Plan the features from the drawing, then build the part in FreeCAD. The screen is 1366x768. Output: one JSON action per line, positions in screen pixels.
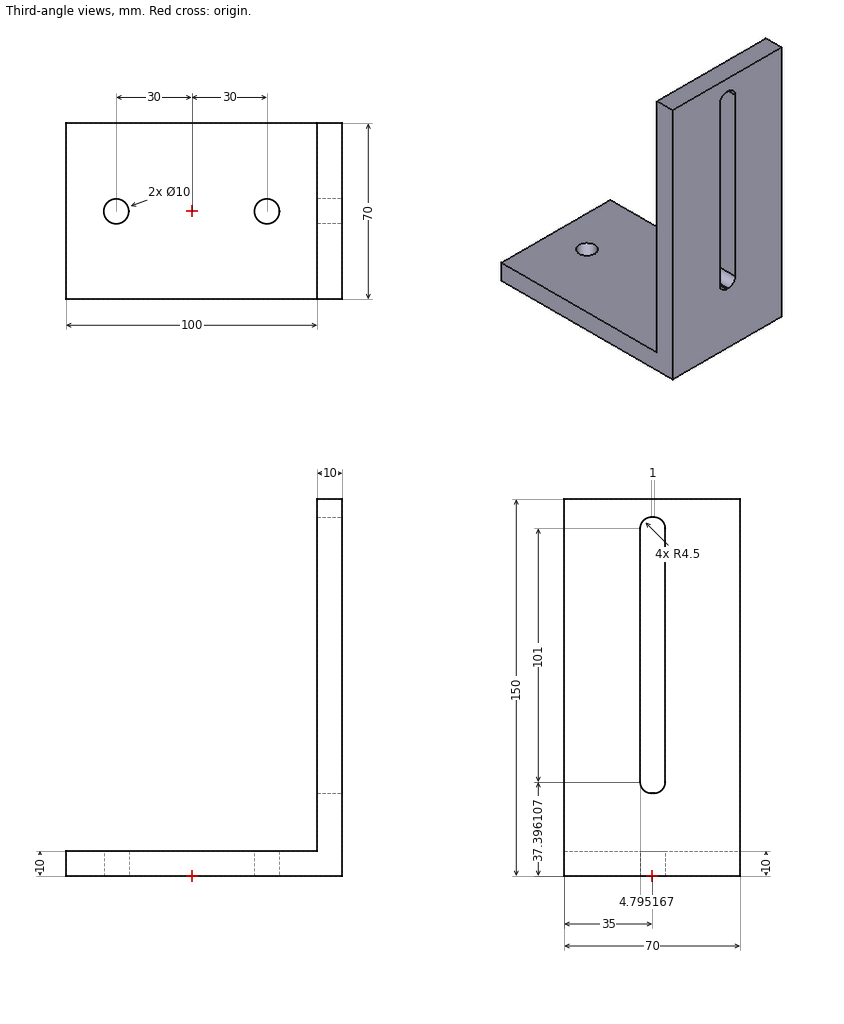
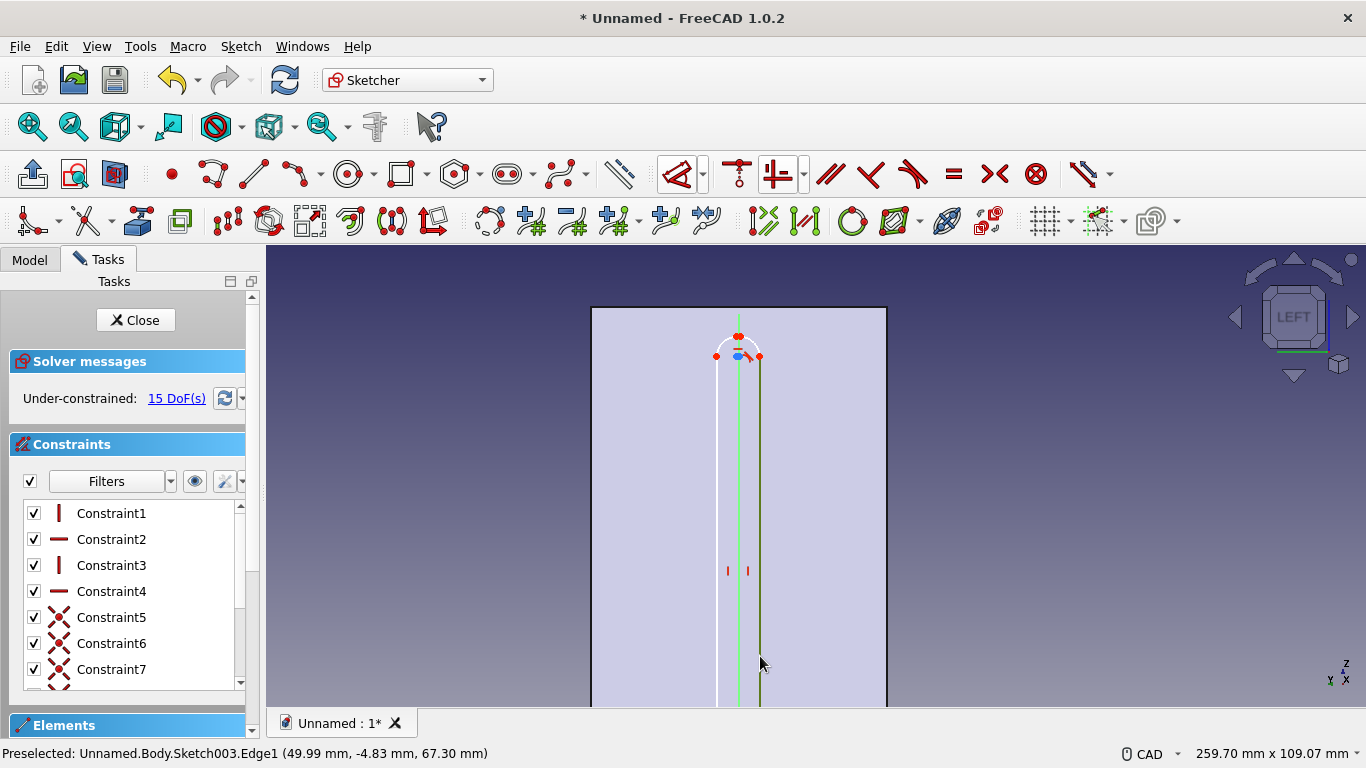
{"action": "scroll", "coordinate": [755, 343], "scroll_direction": "down", "scroll_amount": 4}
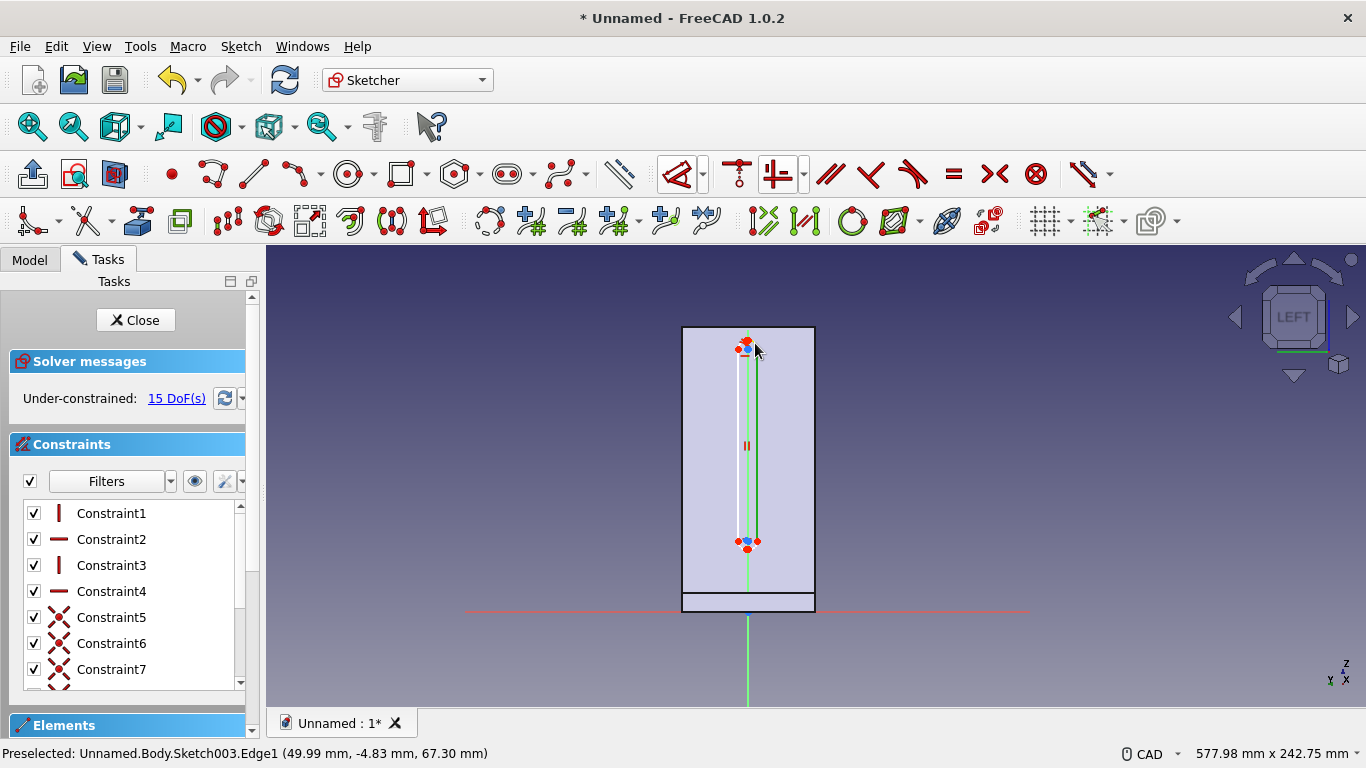
{"action": "scroll", "coordinate": [755, 547], "scroll_direction": "up", "scroll_amount": 4}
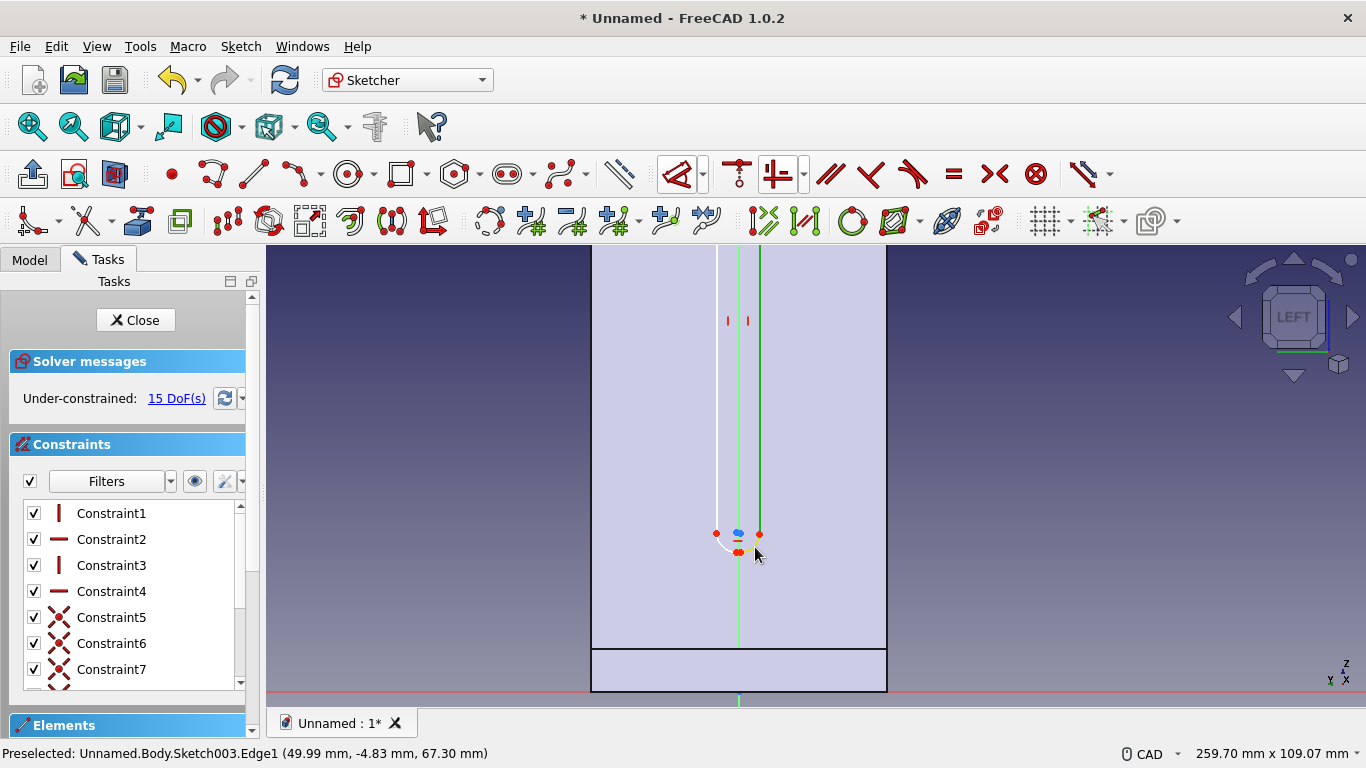
{"action": "left_click", "coordinate": [754, 547]}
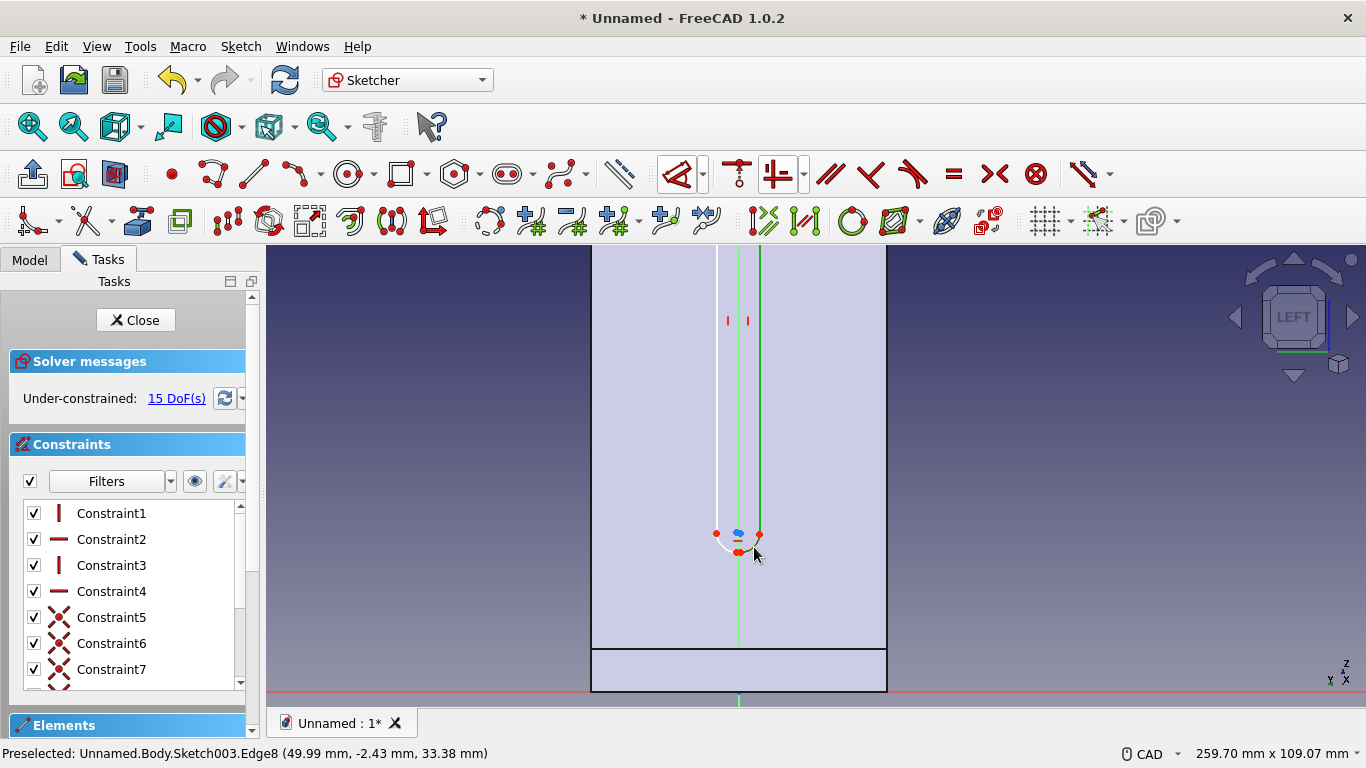
{"action": "left_click", "coordinate": [913, 174]}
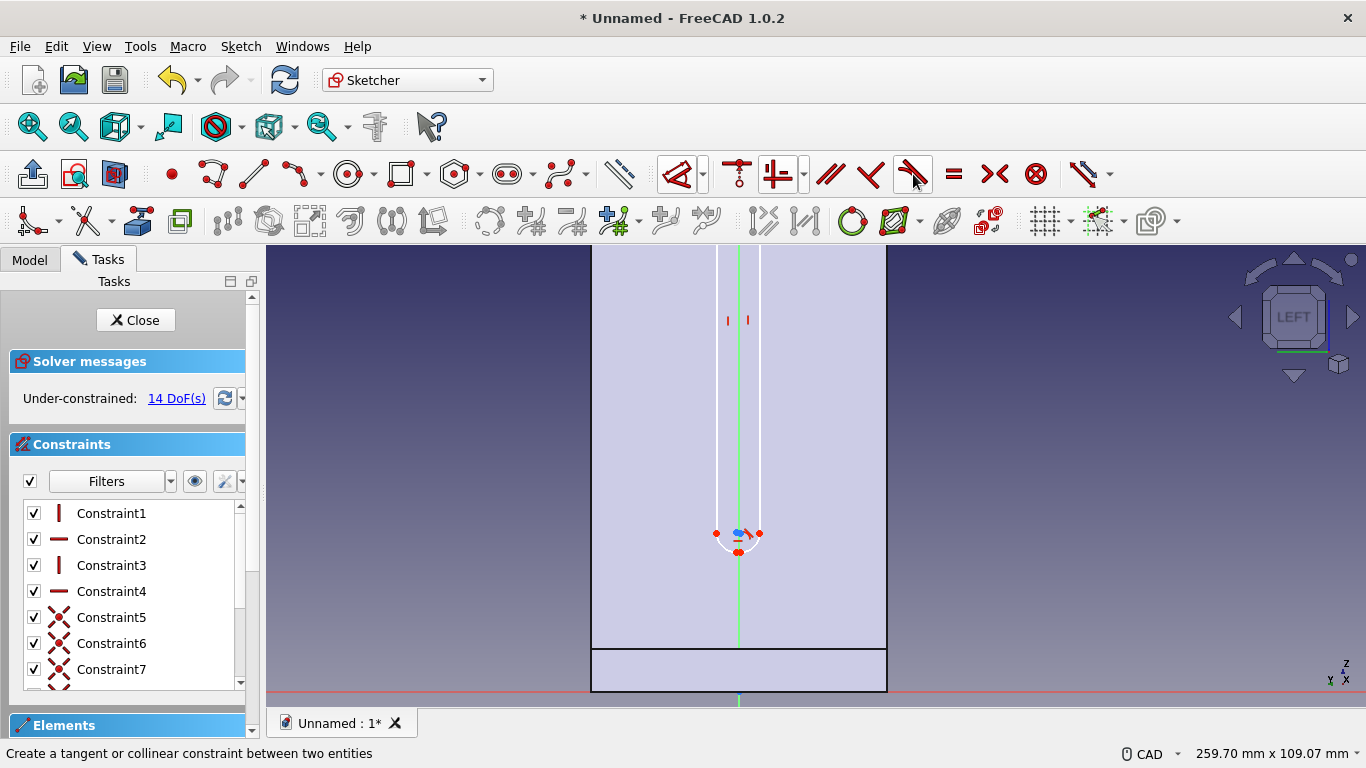
{"action": "scroll", "coordinate": [755, 547], "scroll_direction": "down", "scroll_amount": 4}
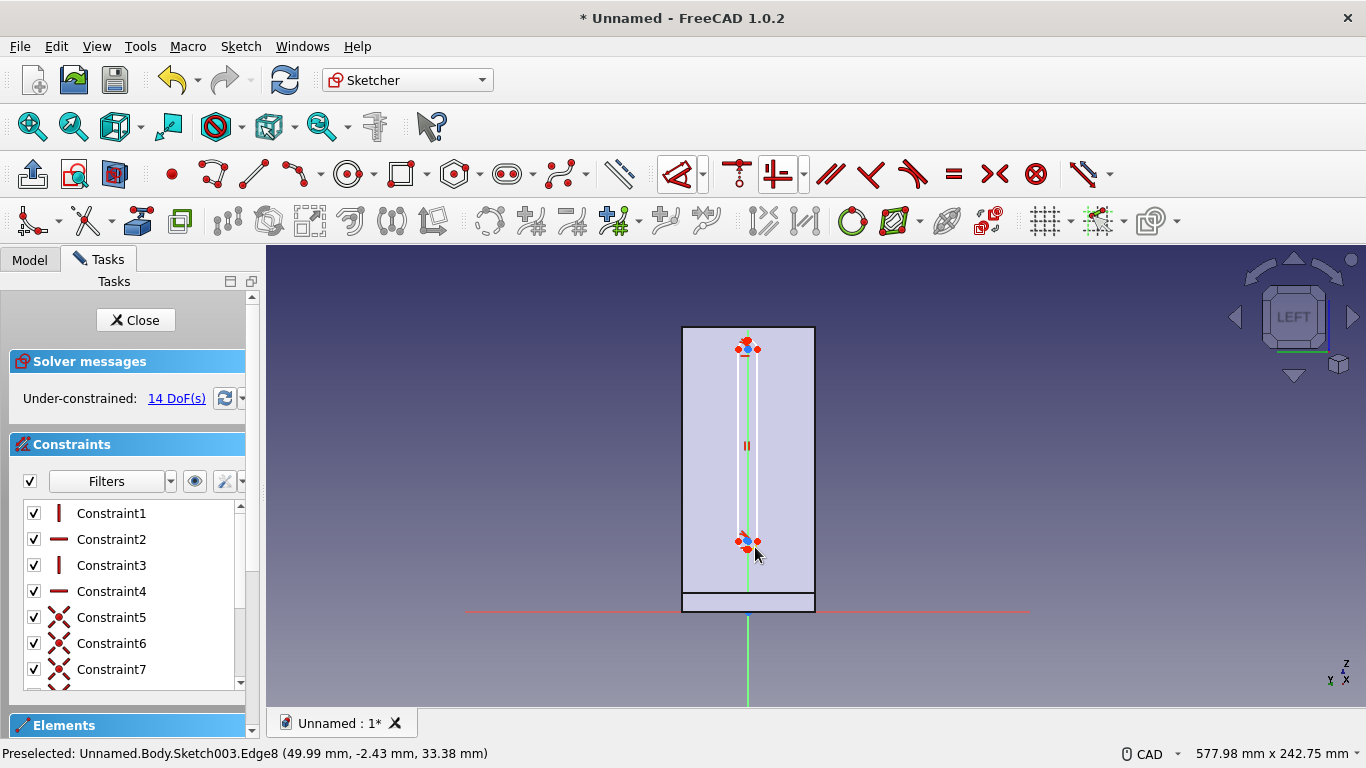
{"action": "scroll", "coordinate": [748, 340], "scroll_direction": "up", "scroll_amount": 14}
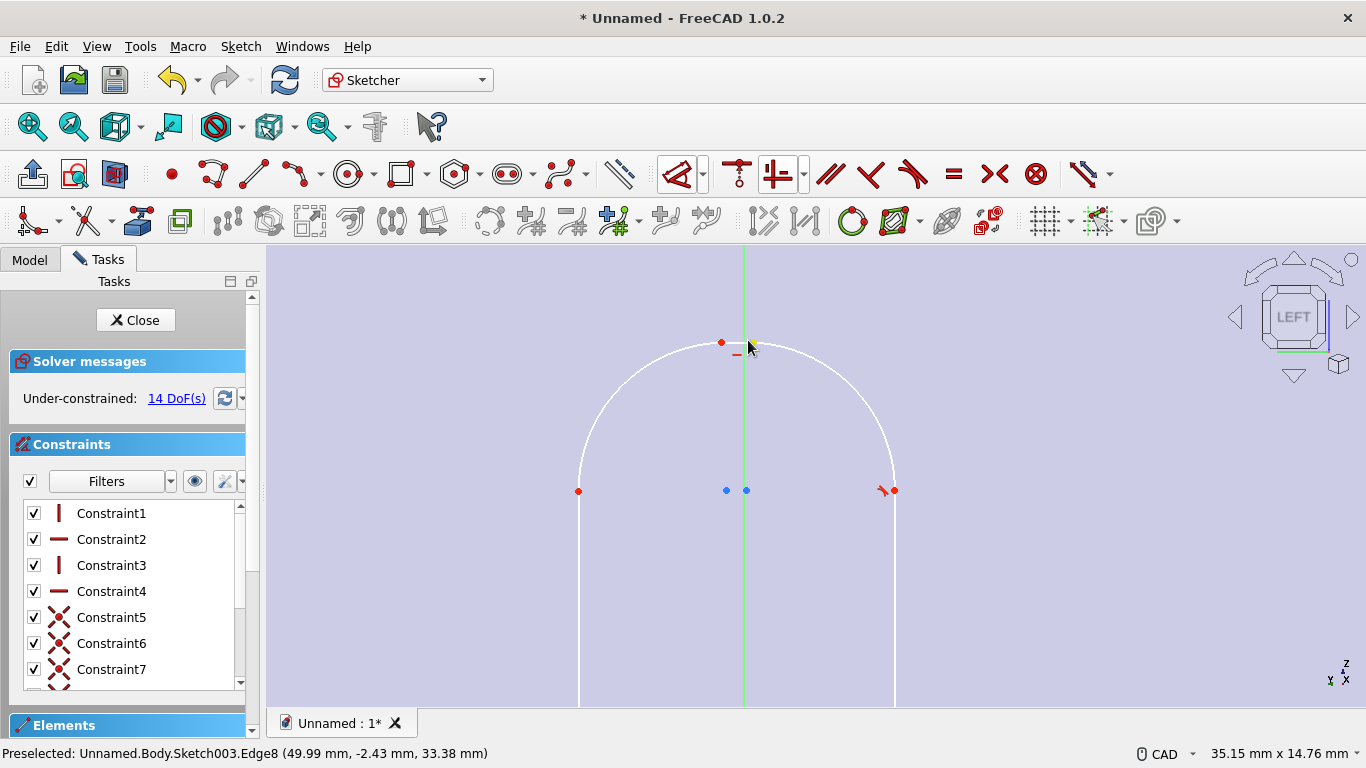
{"action": "left_click", "coordinate": [737, 343]}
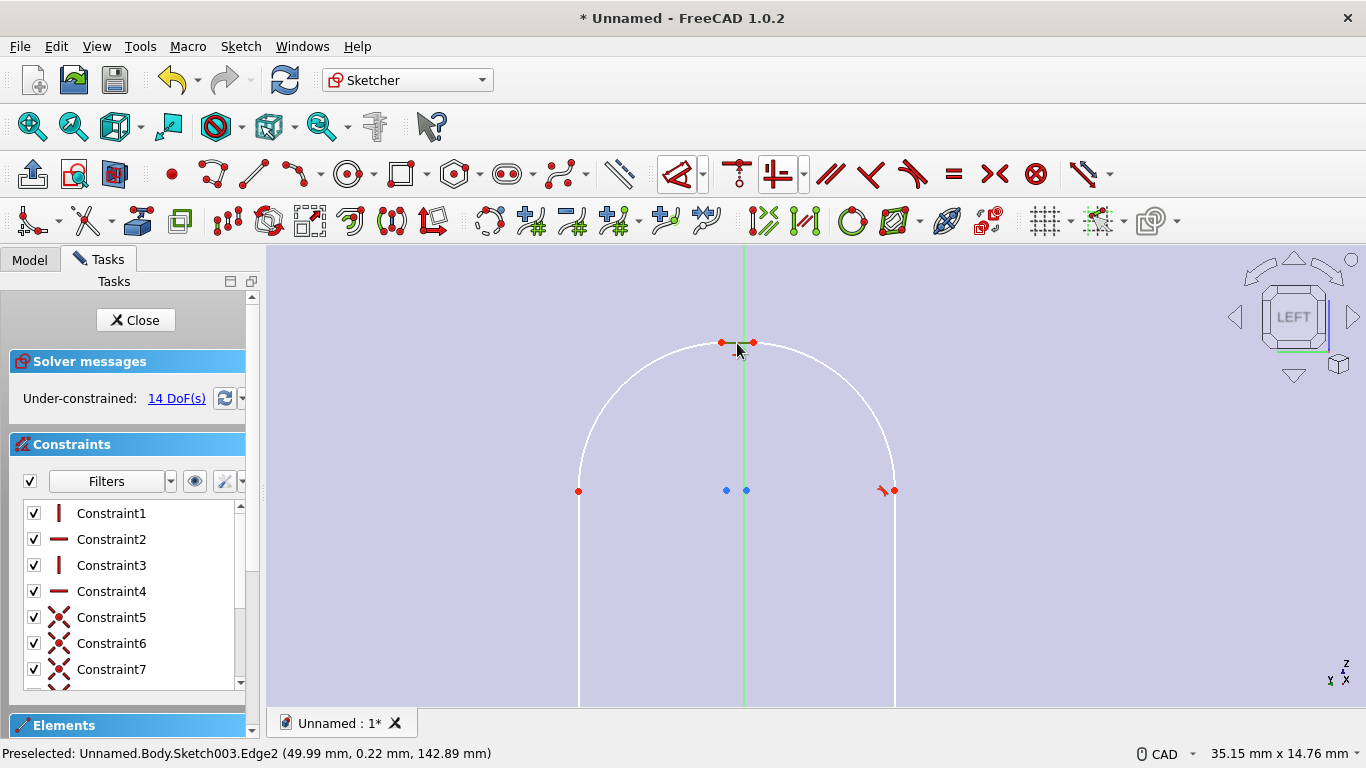
{"action": "scroll", "coordinate": [748, 340], "scroll_direction": "down", "scroll_amount": 14}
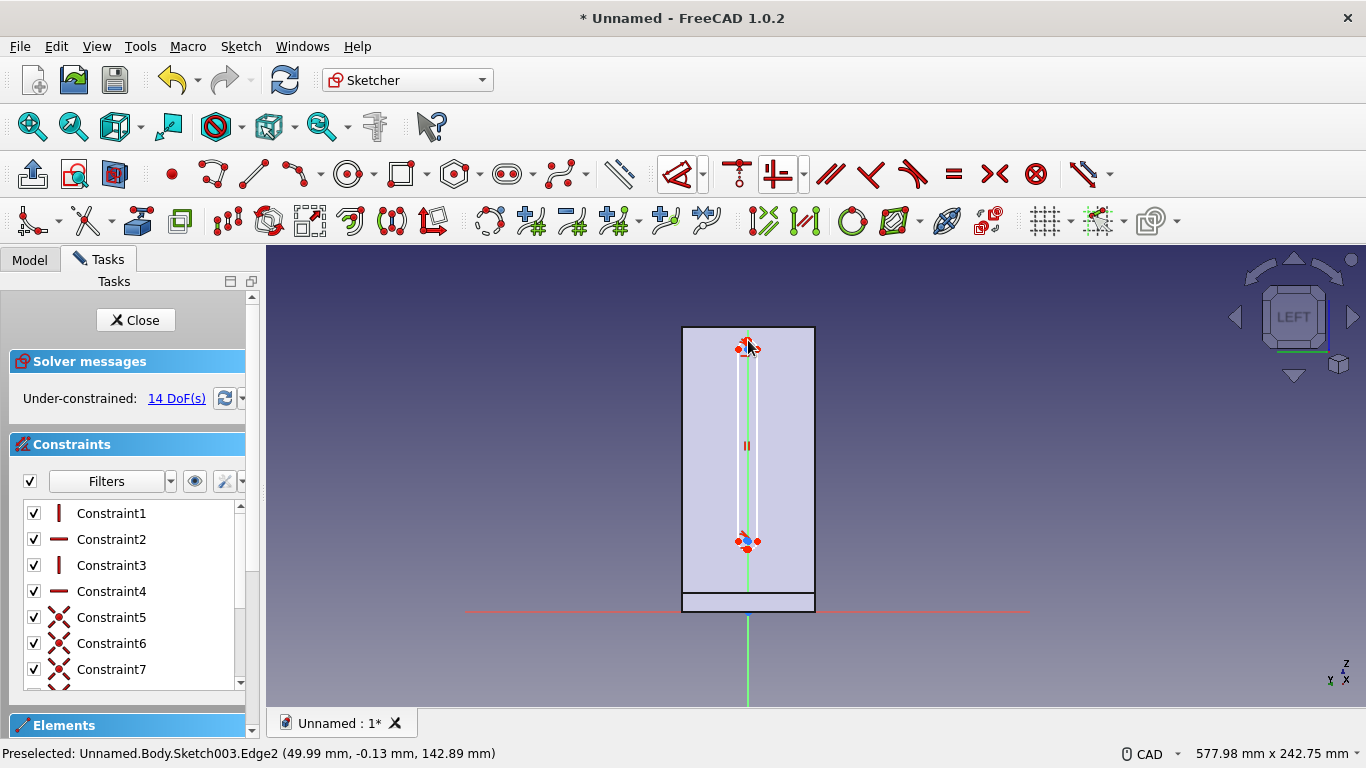
{"action": "scroll", "coordinate": [756, 345], "scroll_direction": "up", "scroll_amount": 7}